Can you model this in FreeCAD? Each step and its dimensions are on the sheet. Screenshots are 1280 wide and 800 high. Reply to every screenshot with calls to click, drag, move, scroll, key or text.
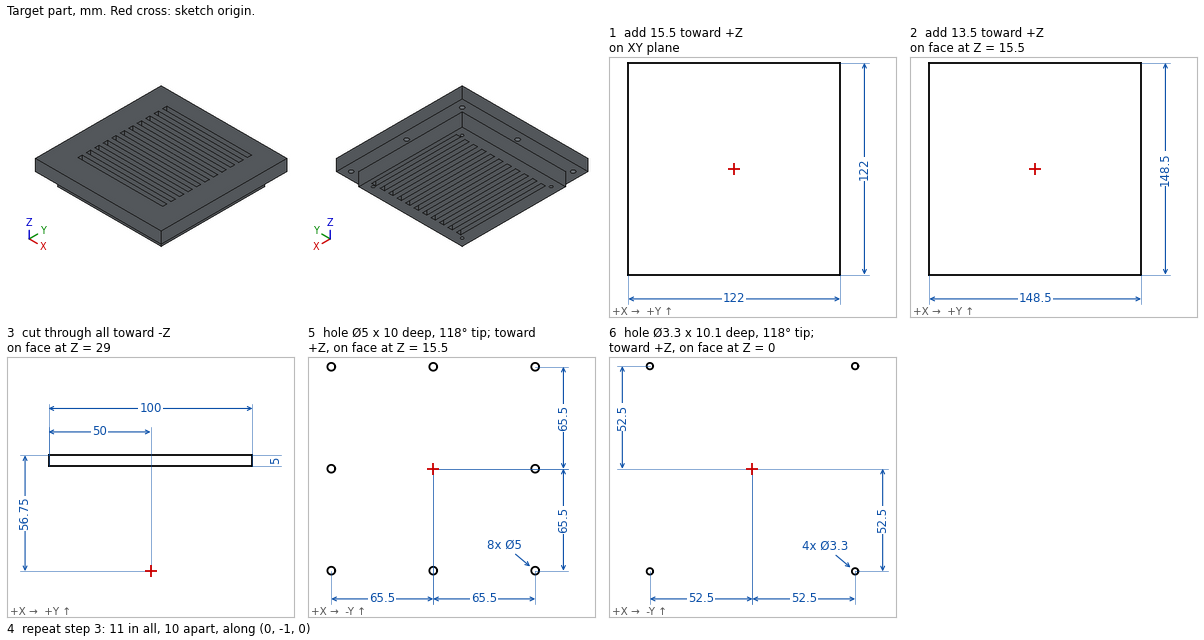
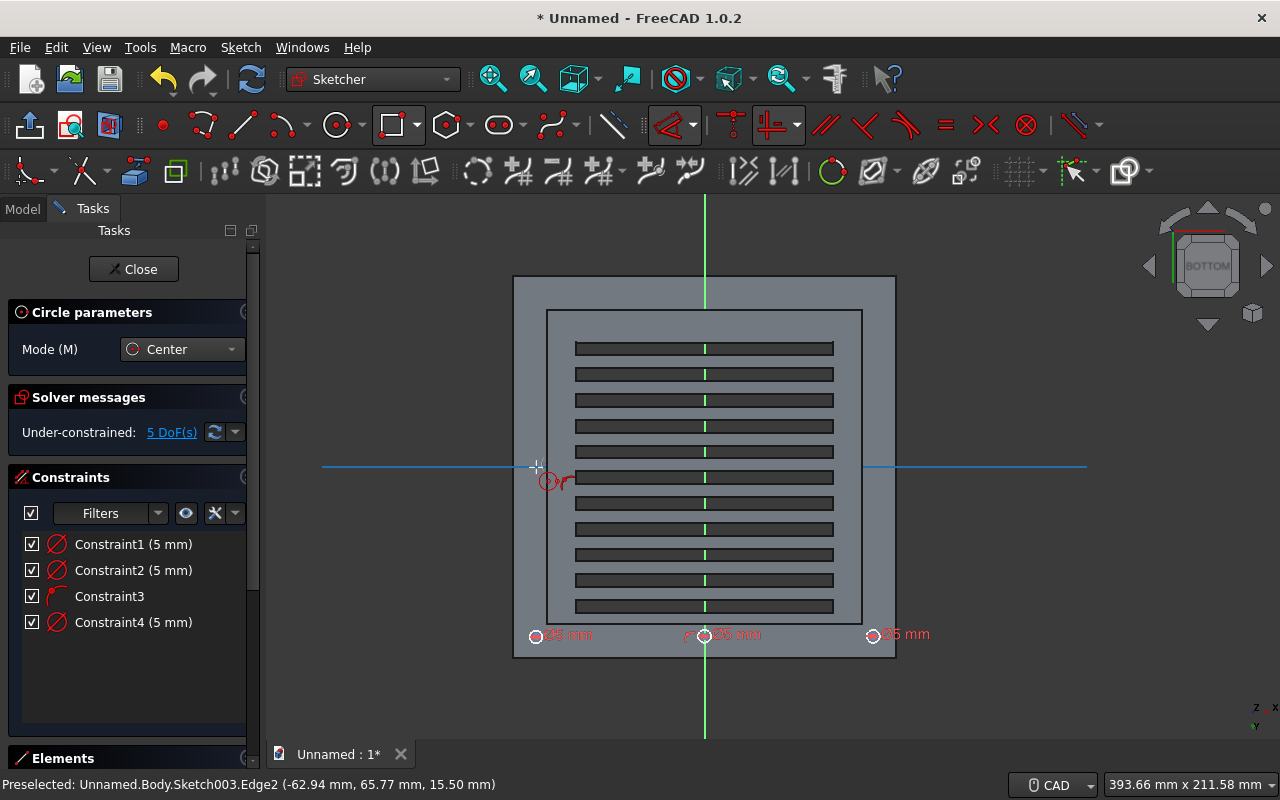
click(536, 467)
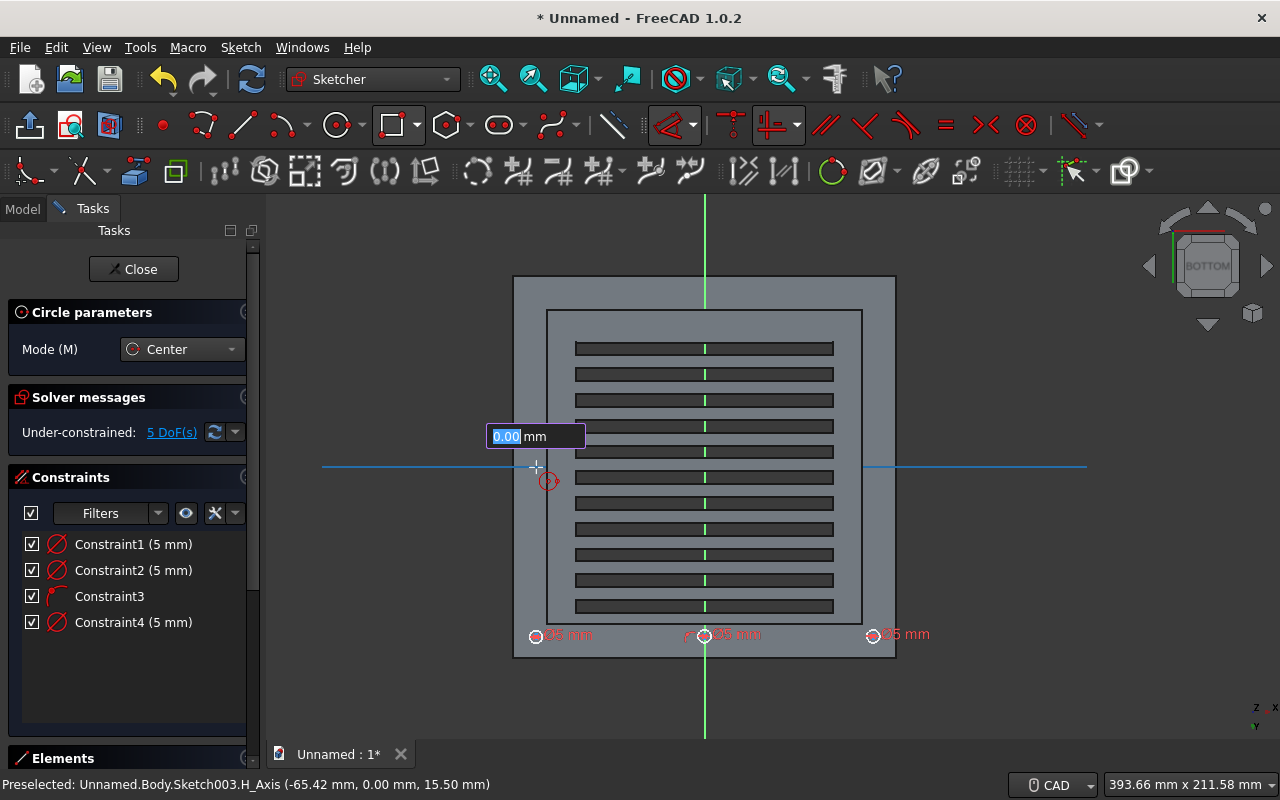
scroll(534, 473, up, 5)
move(532, 472)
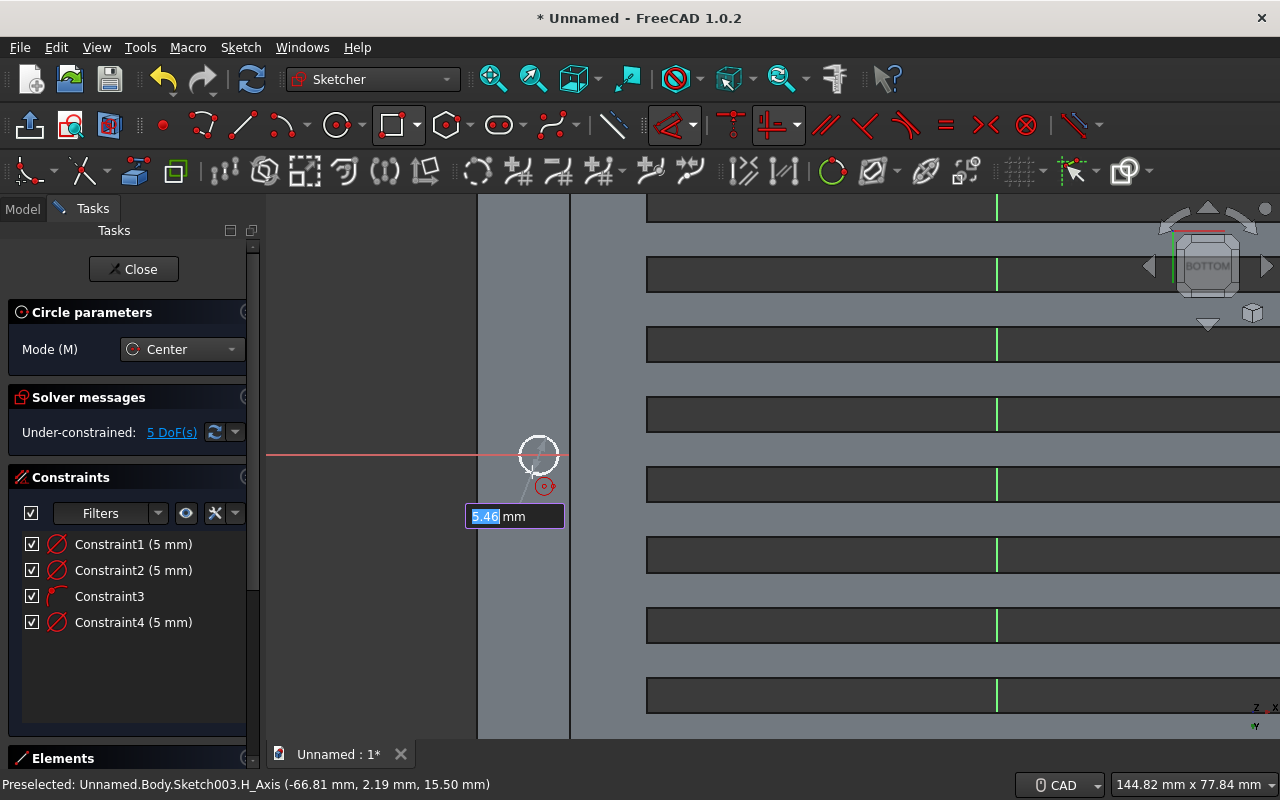
text(5)
key(Return)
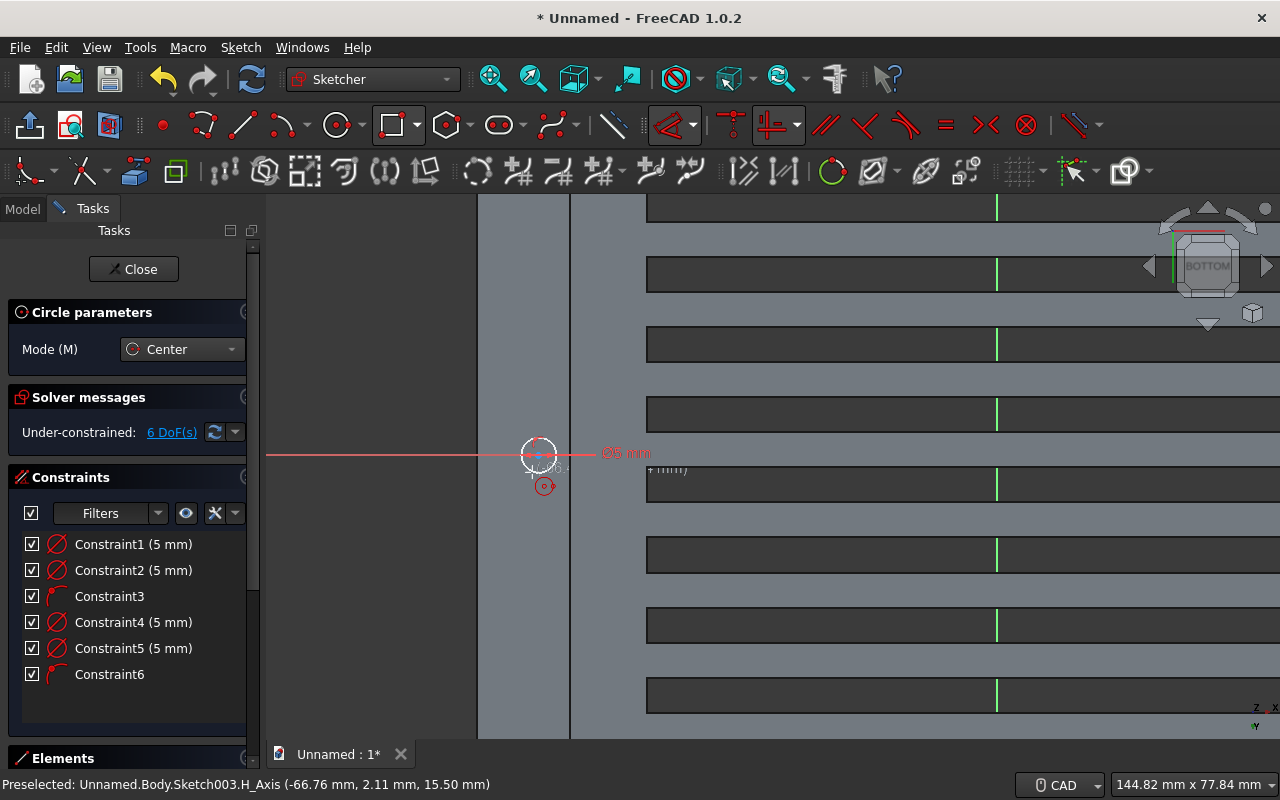
scroll(534, 473, down, 5)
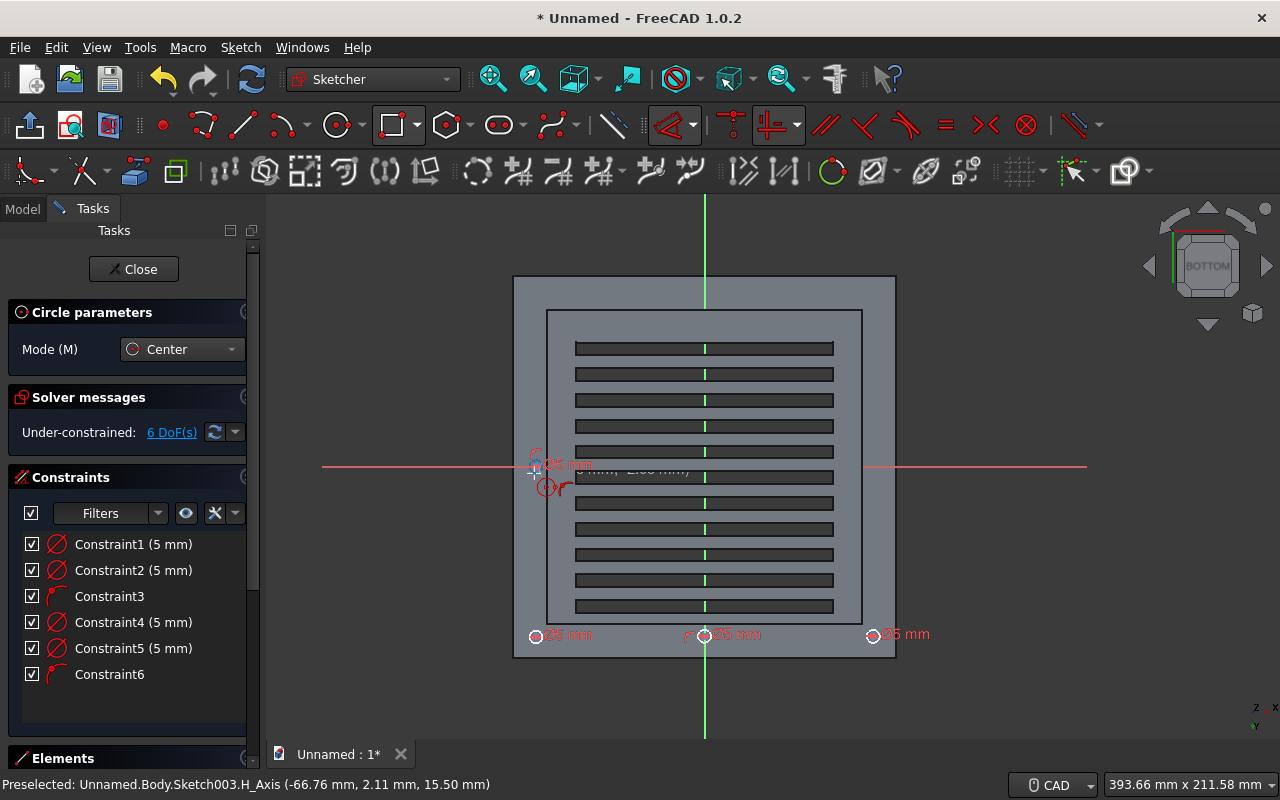
scroll(873, 467, up, 7)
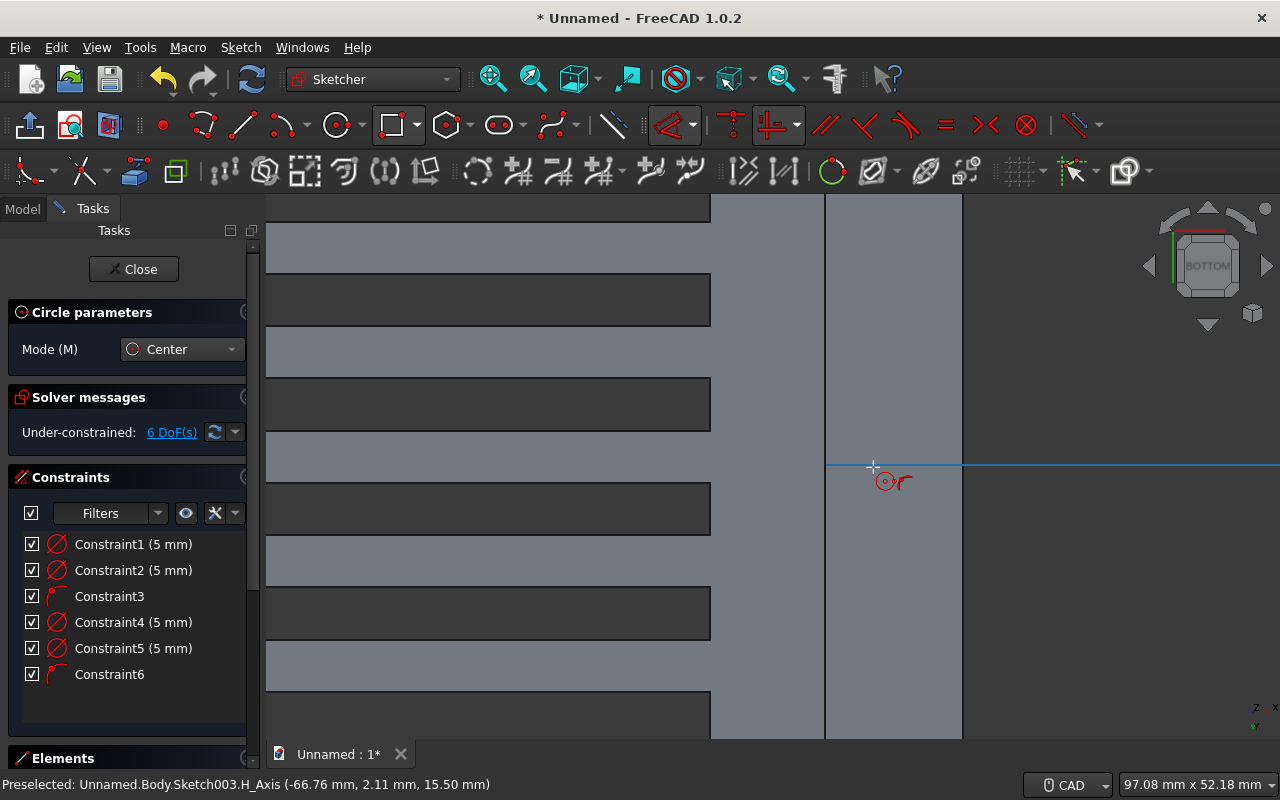
scroll(874, 467, down, 7)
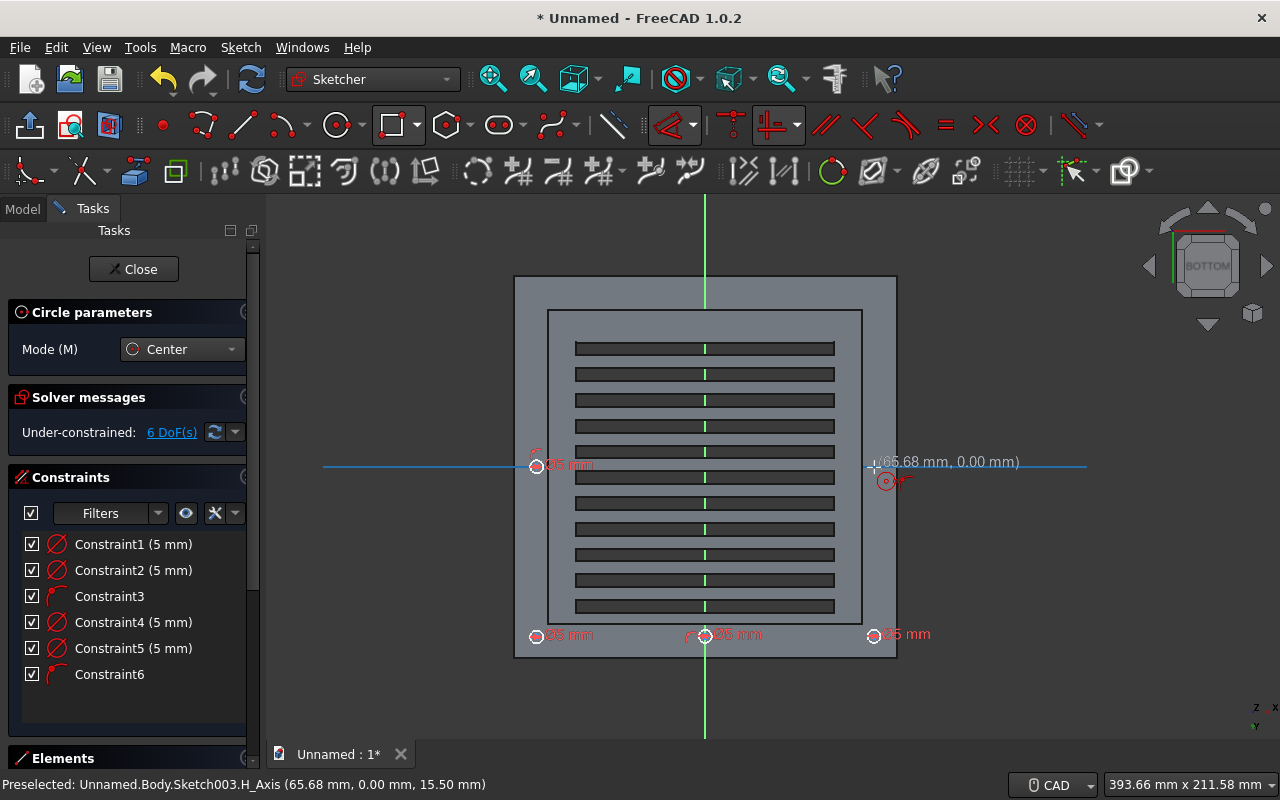
click(874, 467)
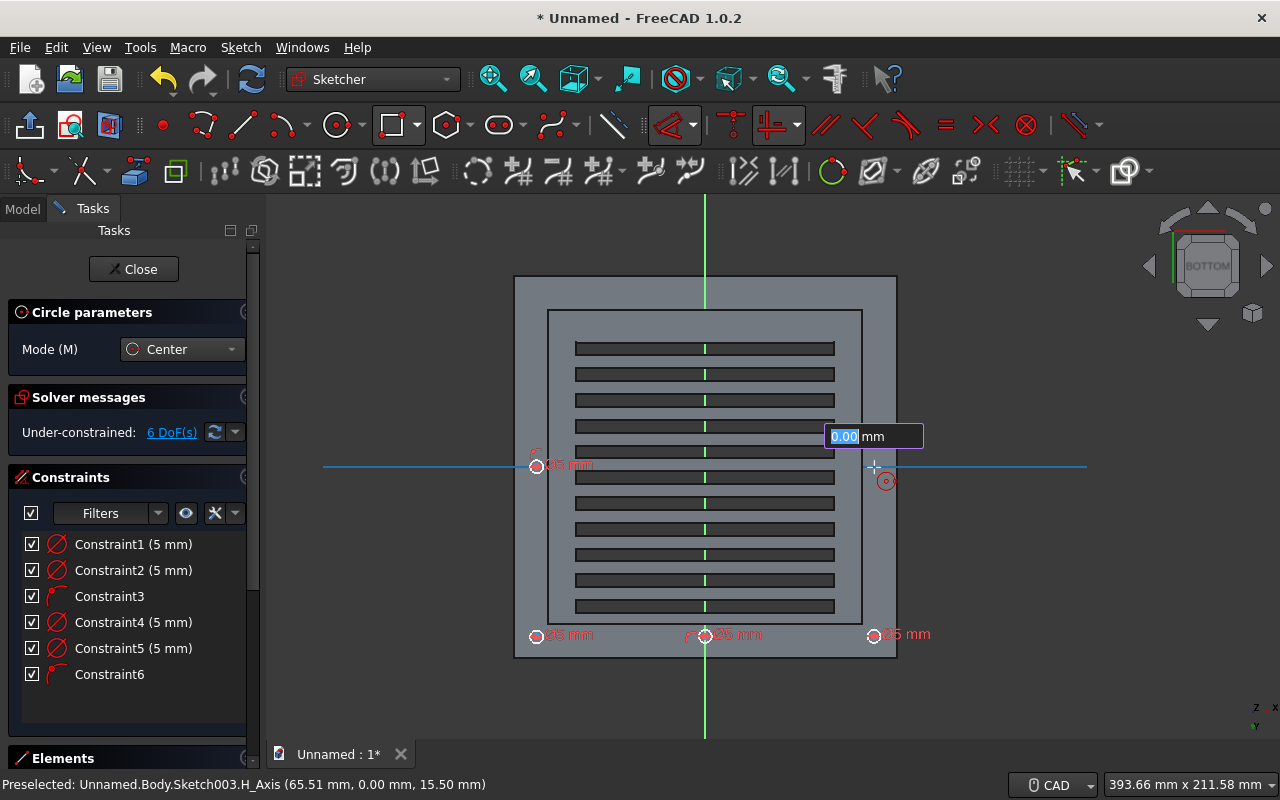
scroll(872, 473, up, 5)
move(870, 472)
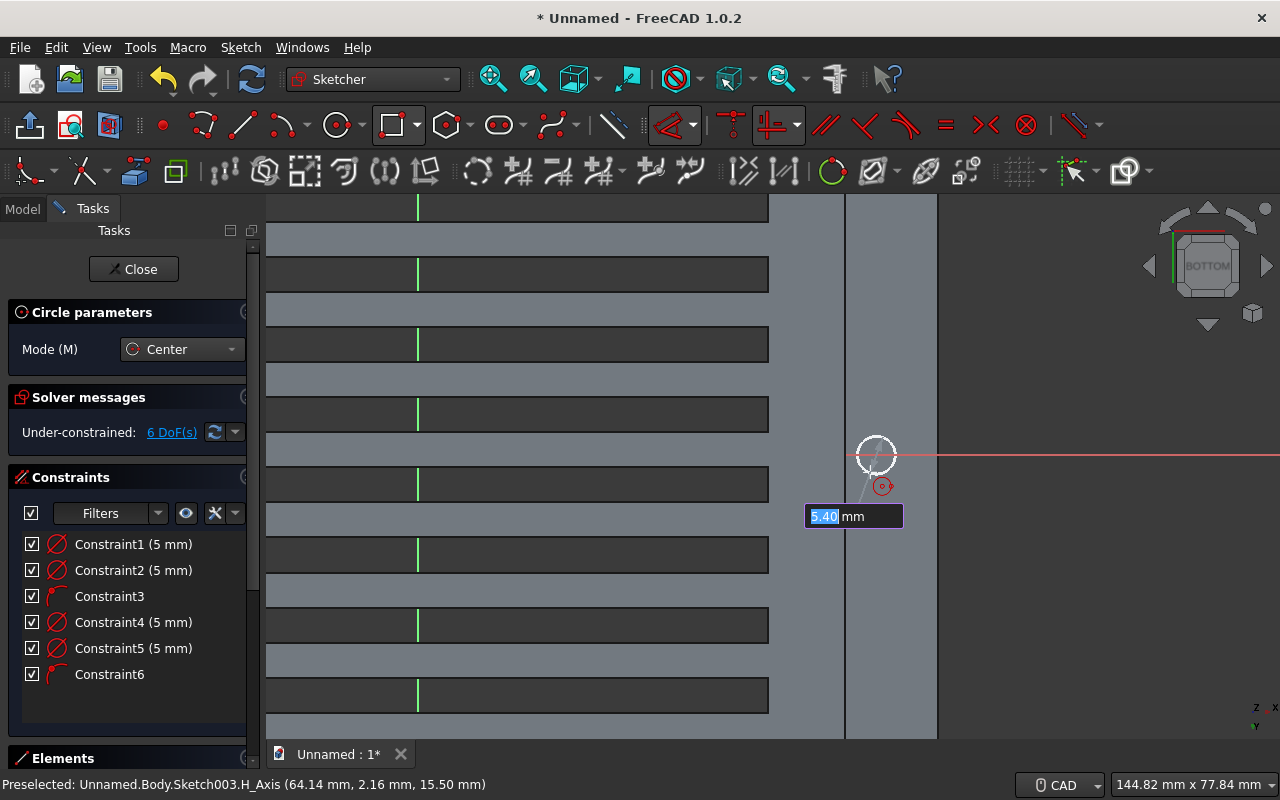
text(5)
key(Return)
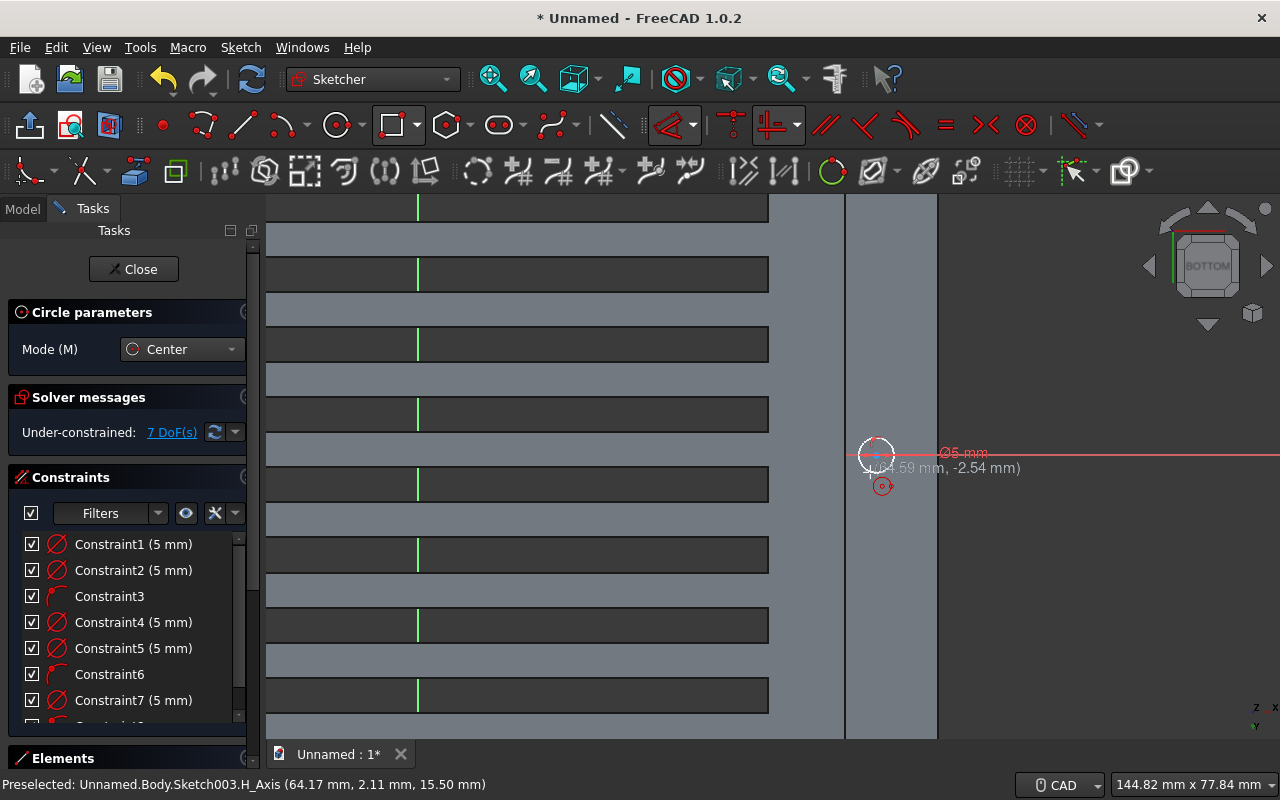
scroll(871, 473, down, 5)